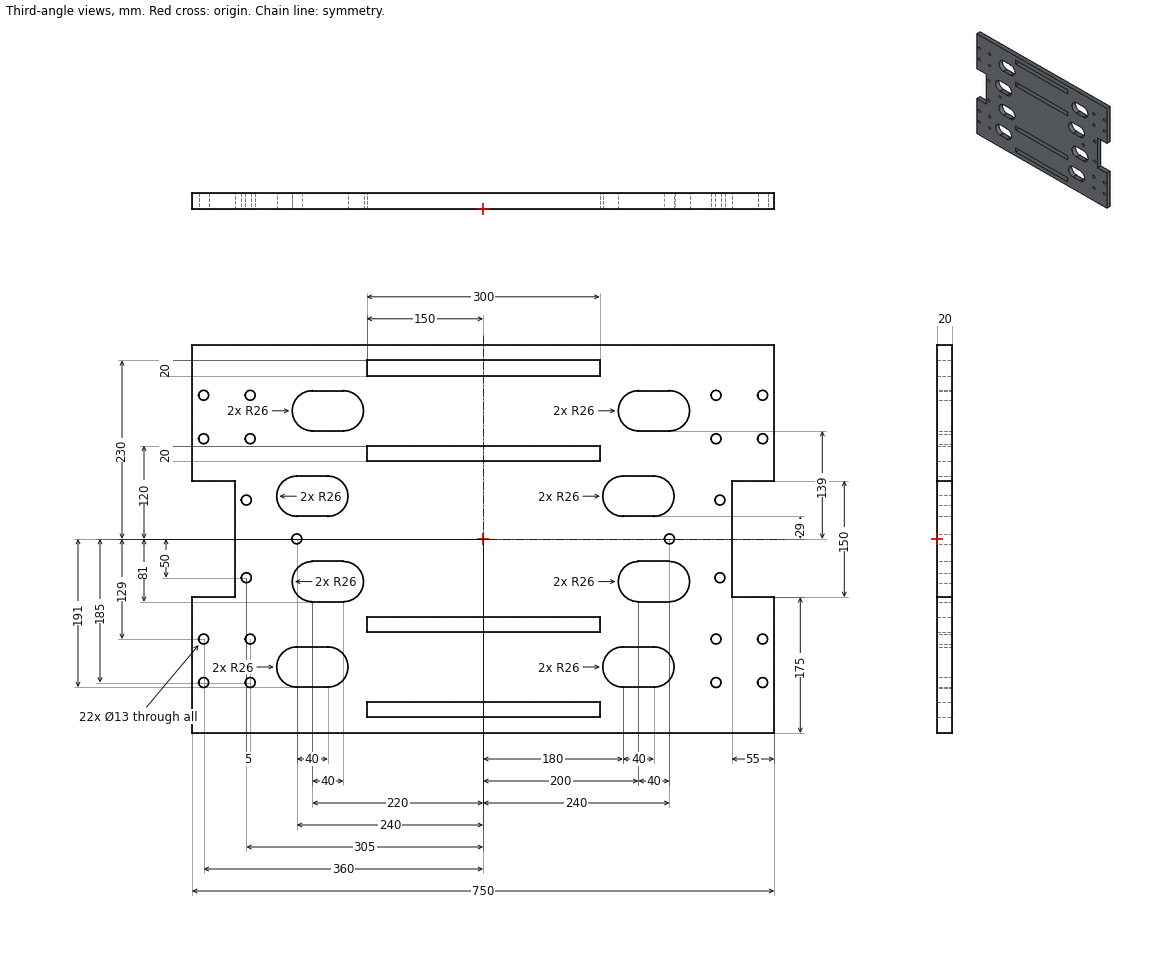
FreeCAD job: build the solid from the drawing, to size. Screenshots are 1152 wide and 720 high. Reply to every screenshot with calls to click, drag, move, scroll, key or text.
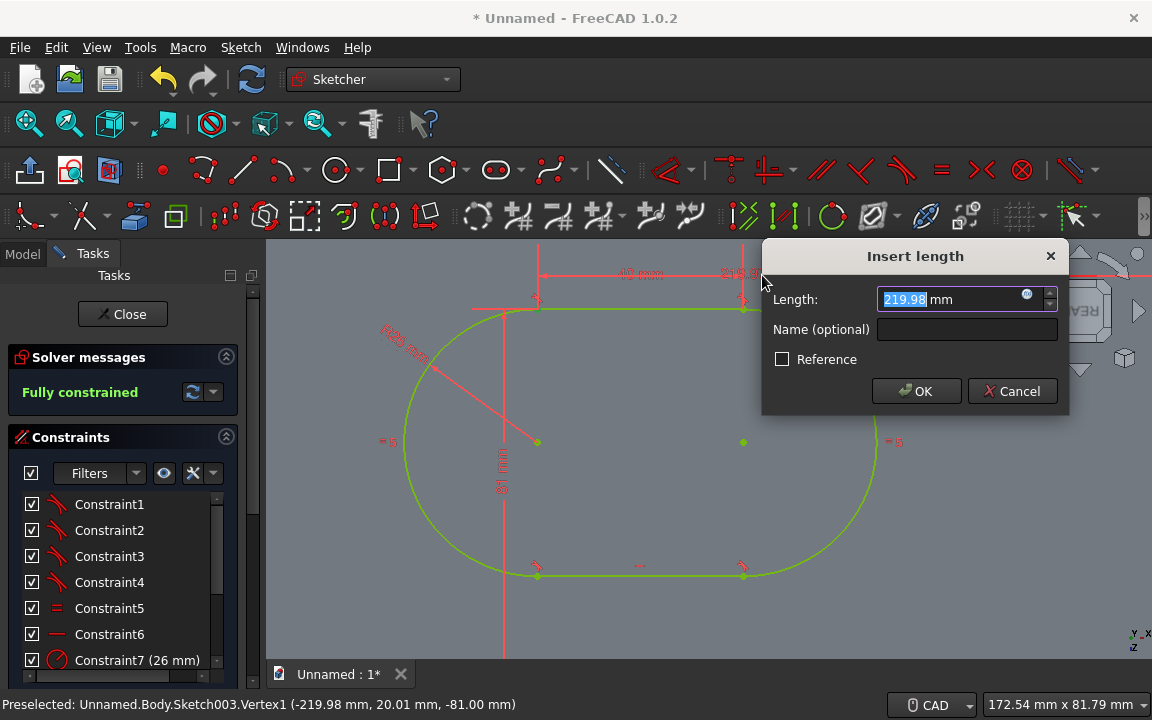
text(220)
key(Return)
key(Escape)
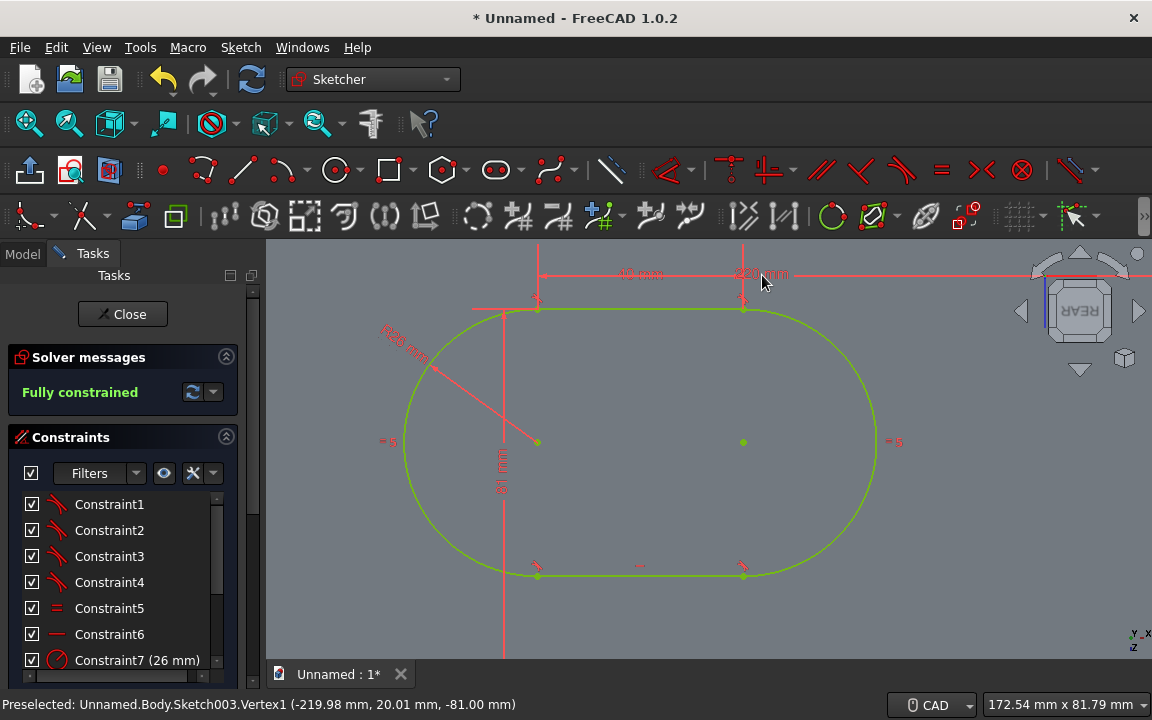
click(123, 314)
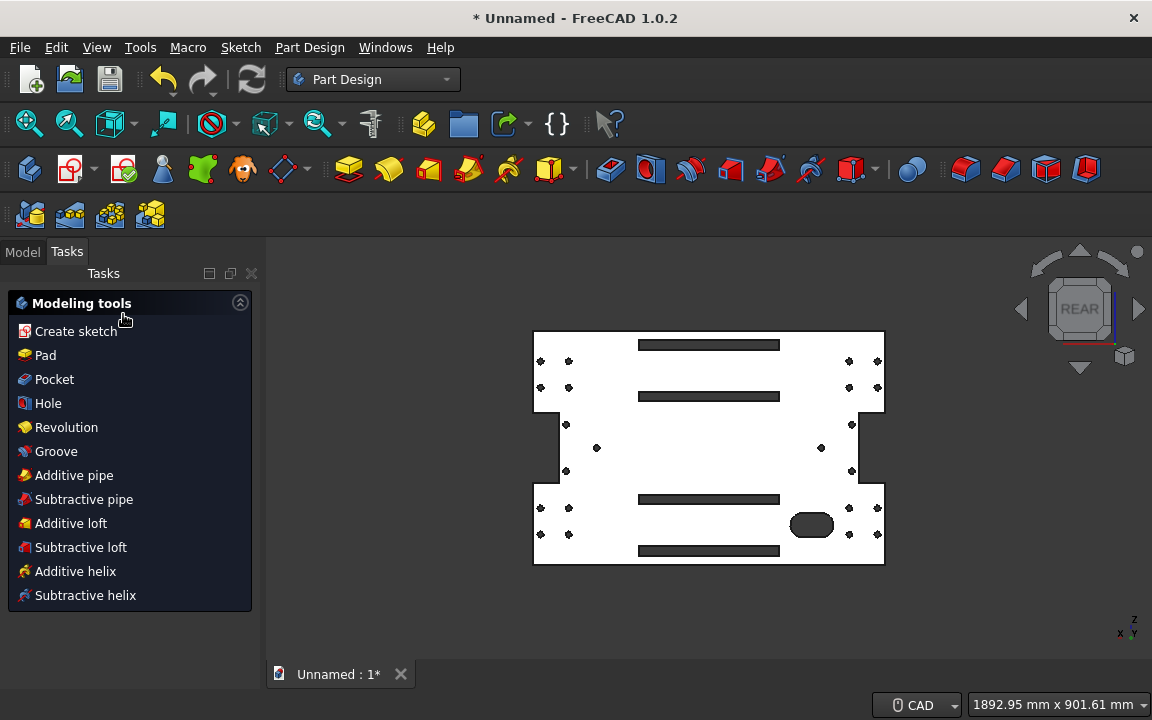
click(612, 170)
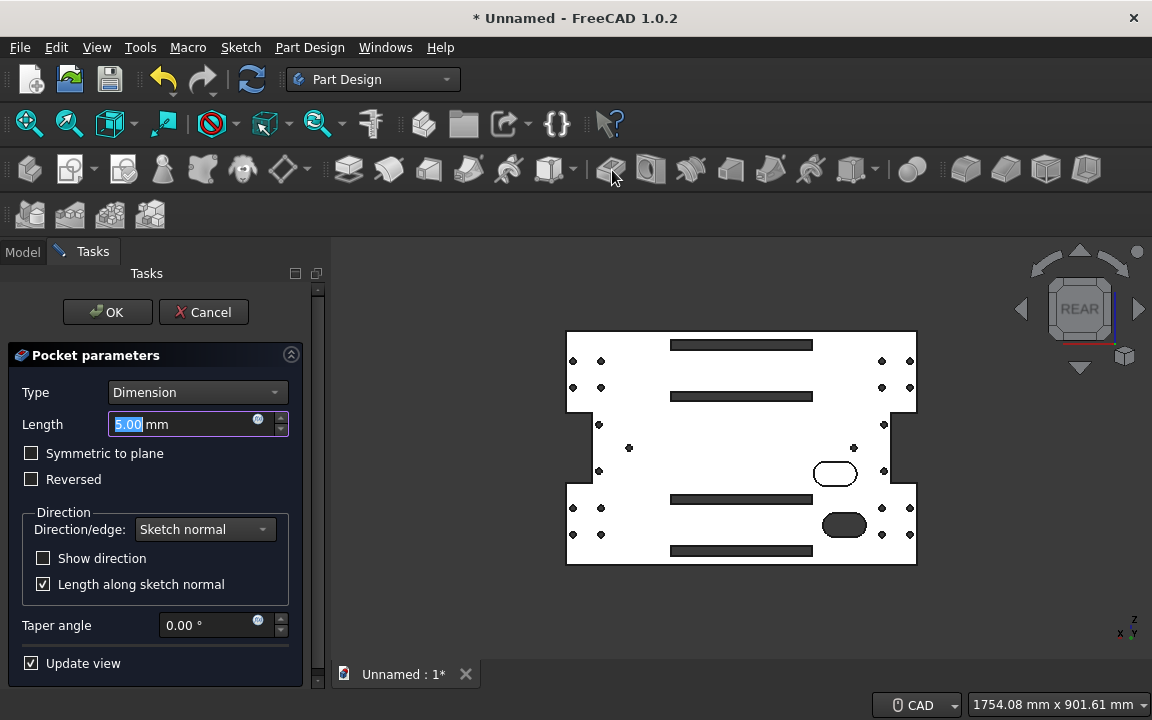
click(198, 392)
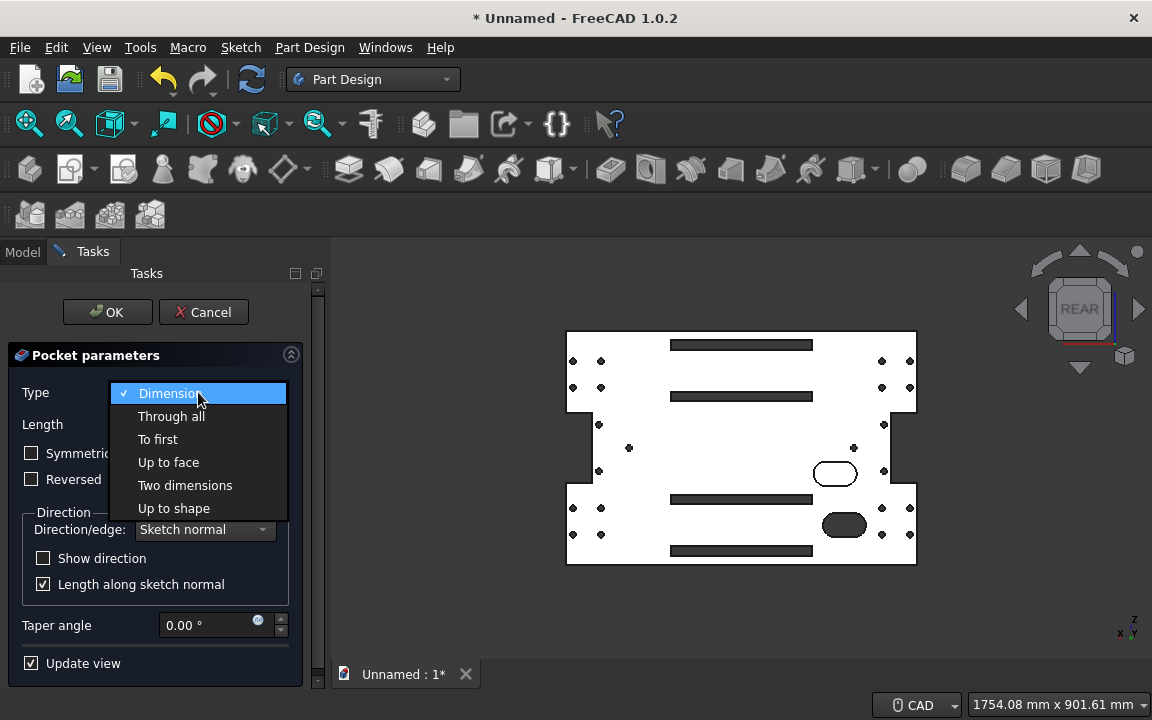
click(198, 440)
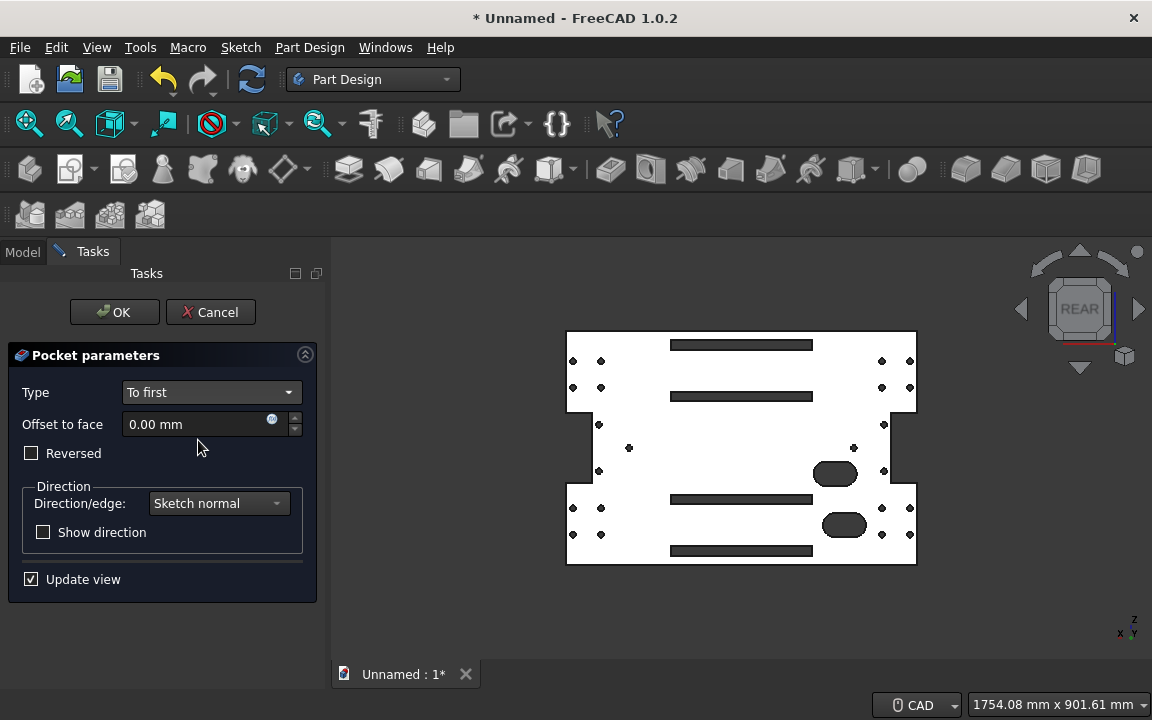
click(115, 312)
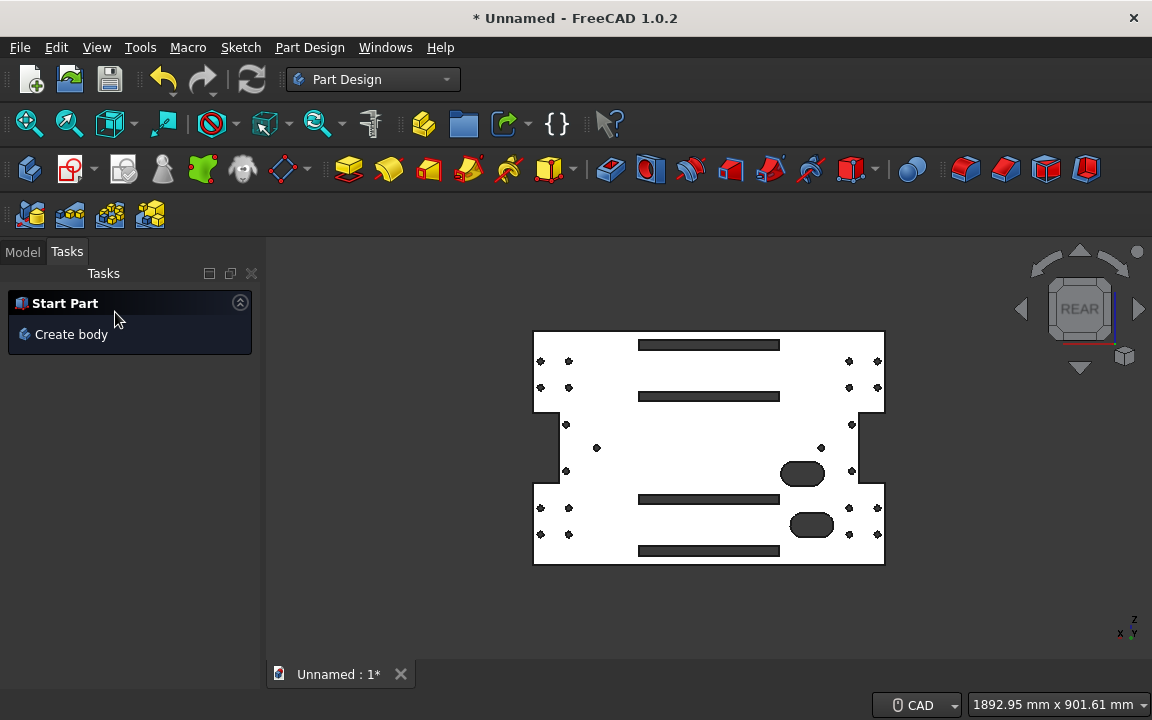
click(659, 447)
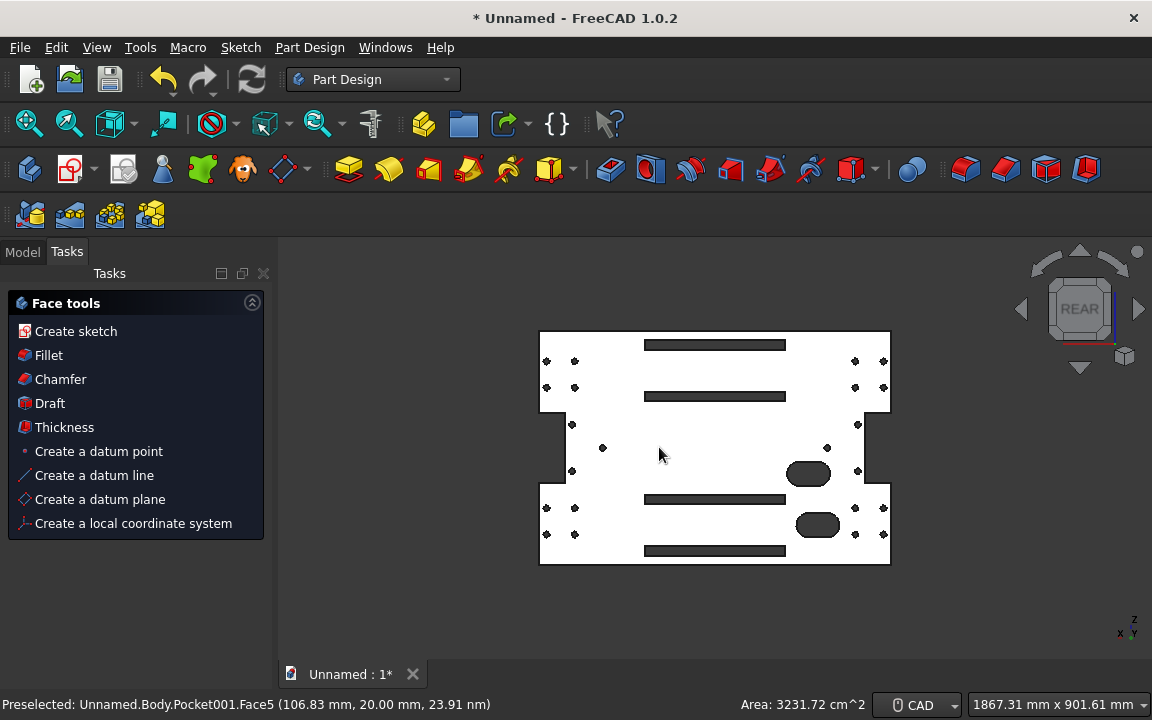
click(70, 170)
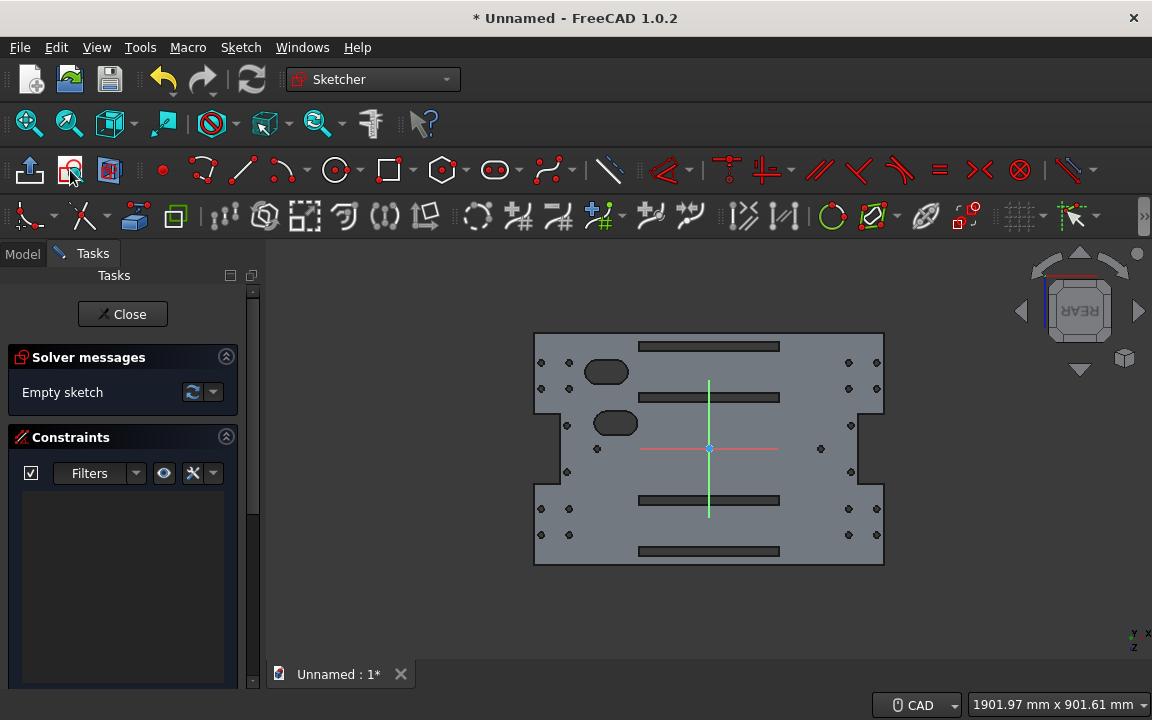
scroll(818, 364, up, 12)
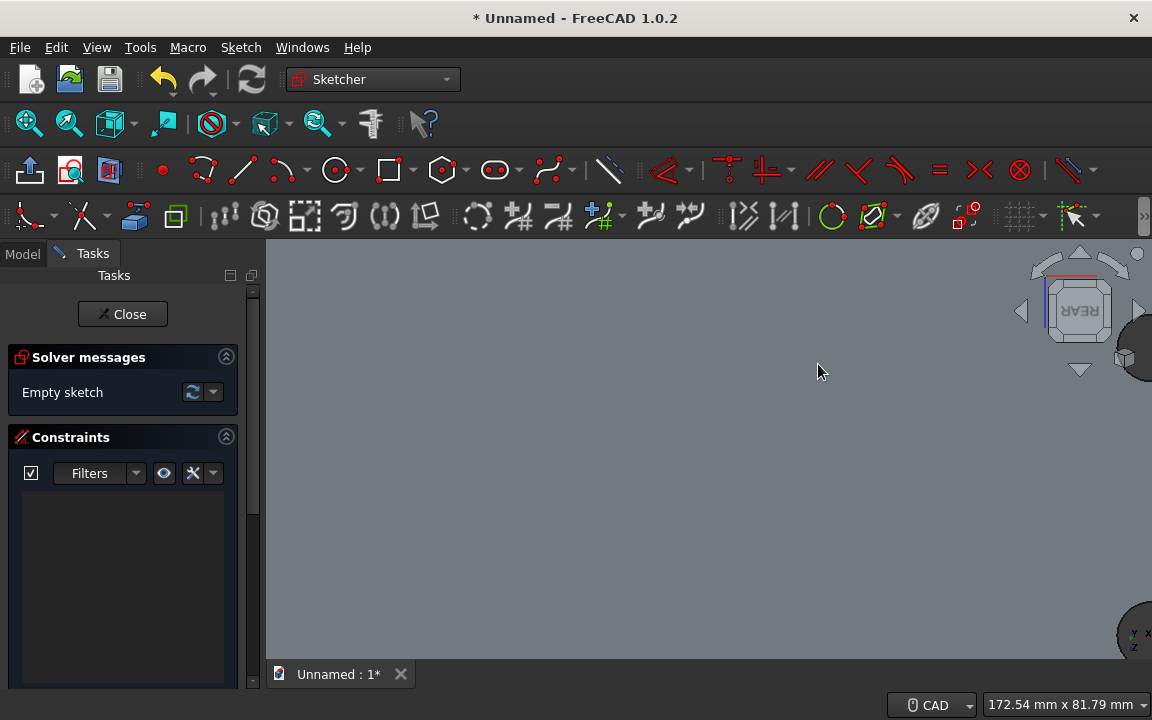
click(496, 170)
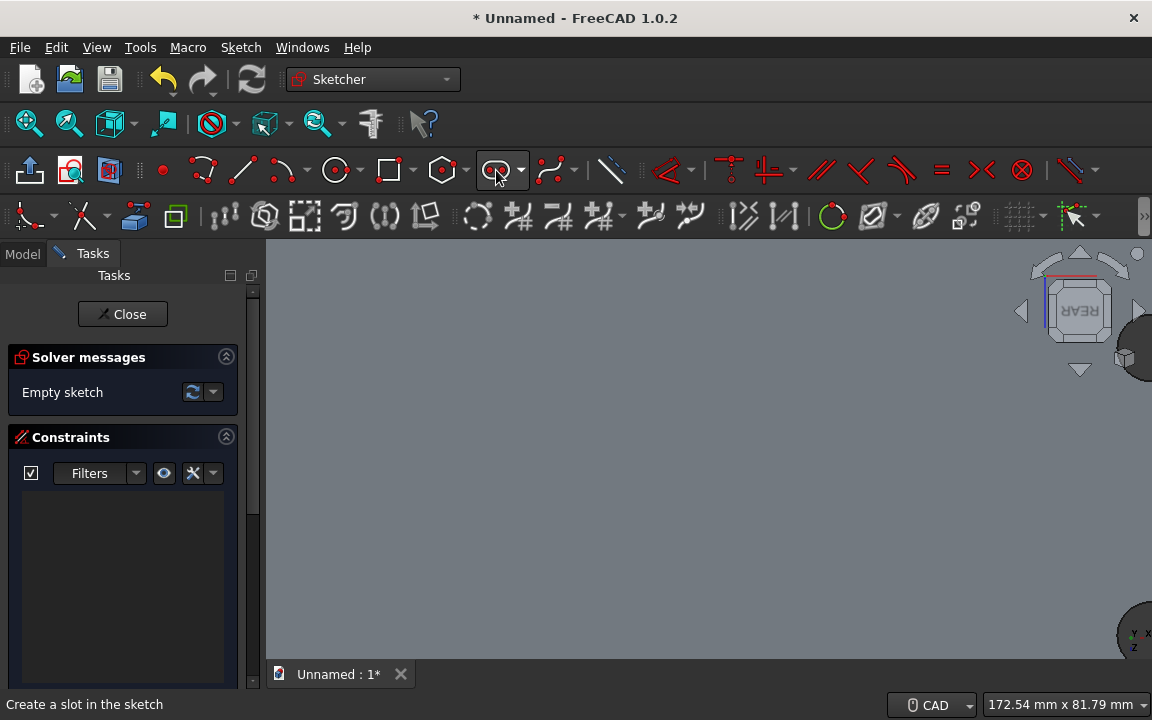
click(535, 451)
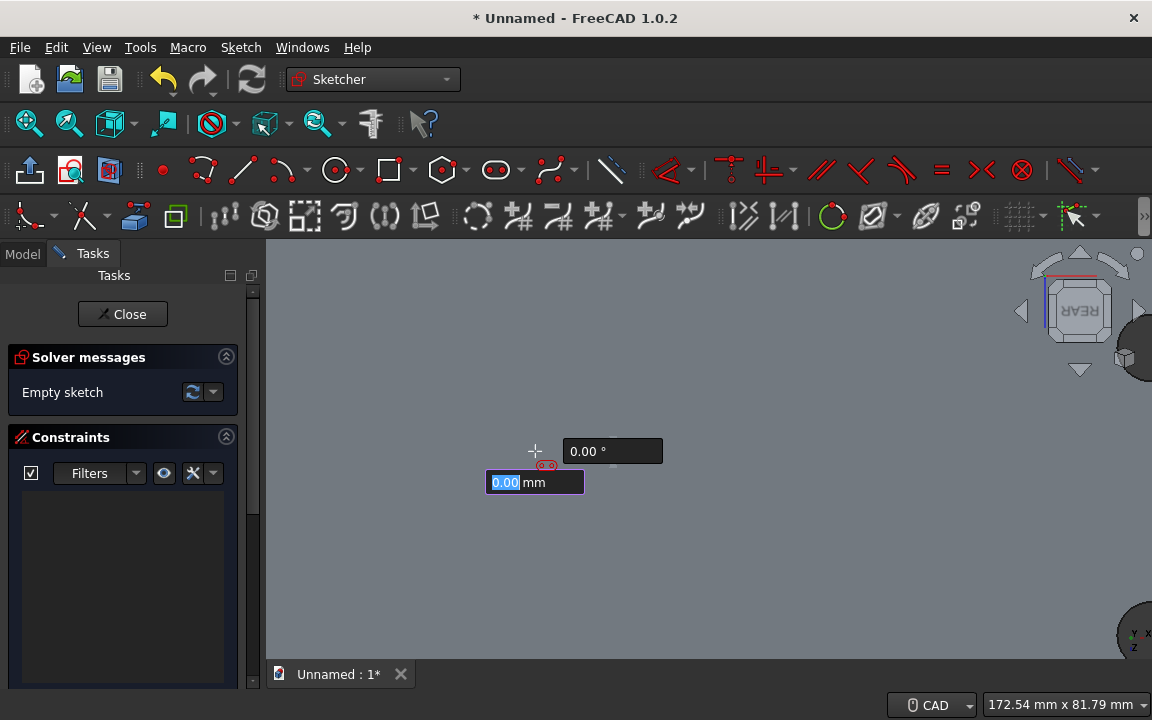
click(740, 451)